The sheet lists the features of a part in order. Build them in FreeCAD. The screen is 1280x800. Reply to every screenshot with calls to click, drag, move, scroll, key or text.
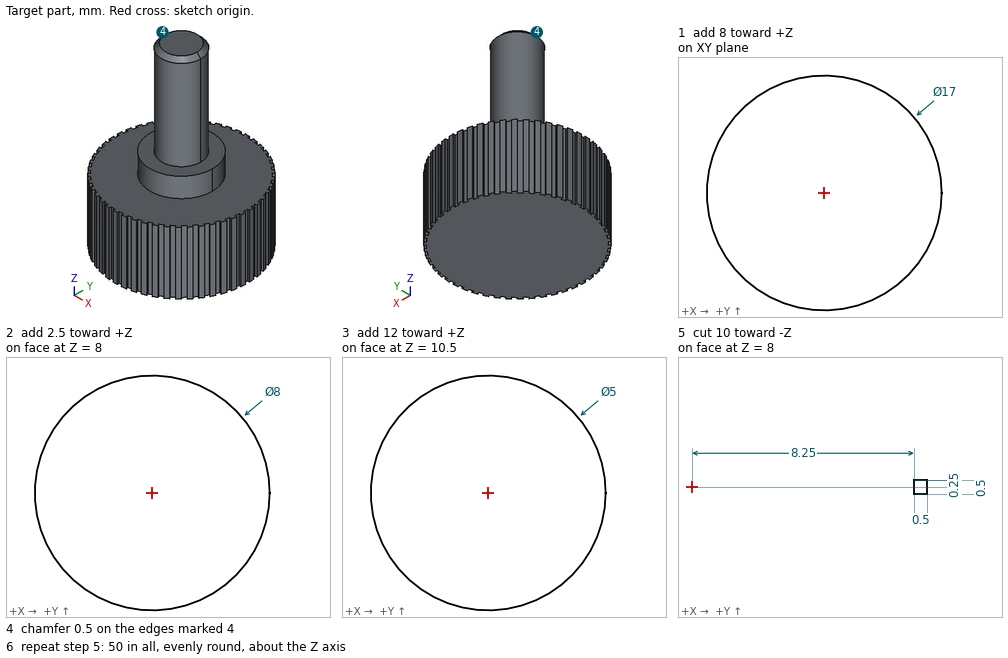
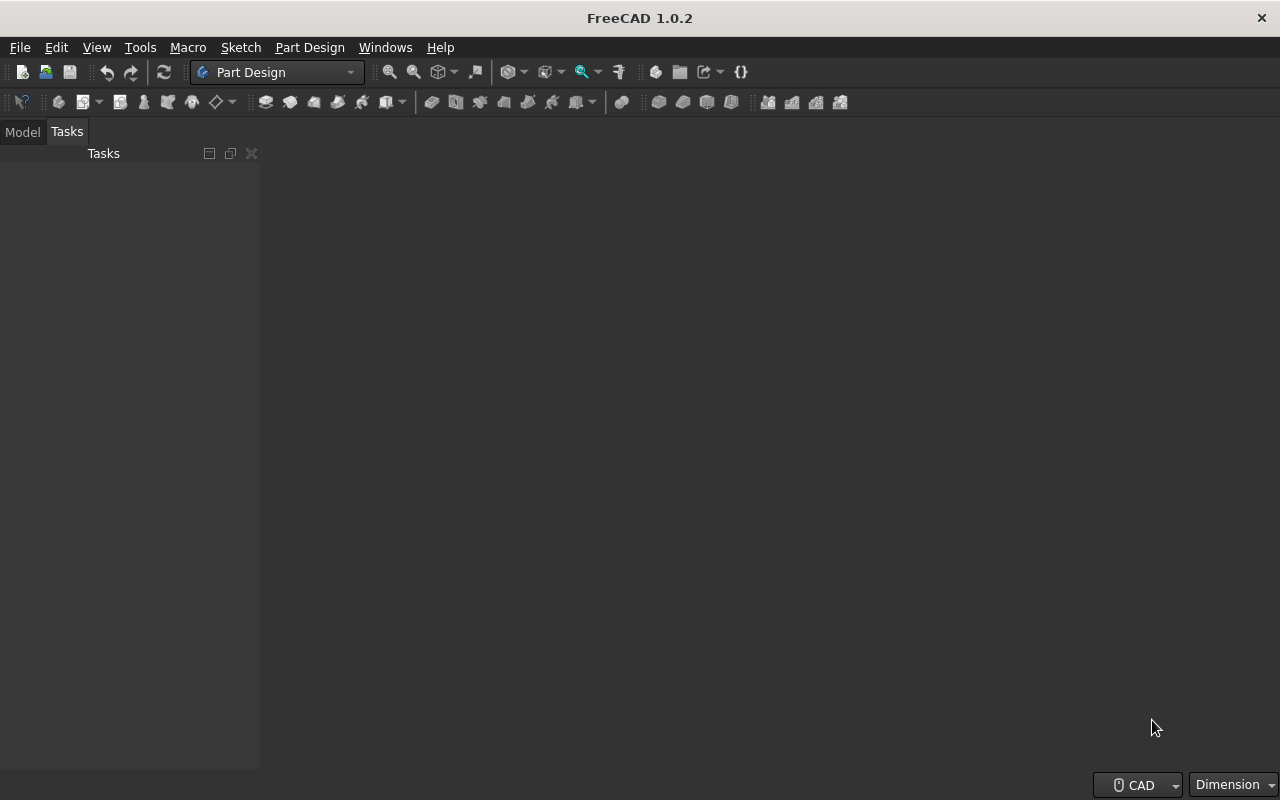
key(ctrl+n)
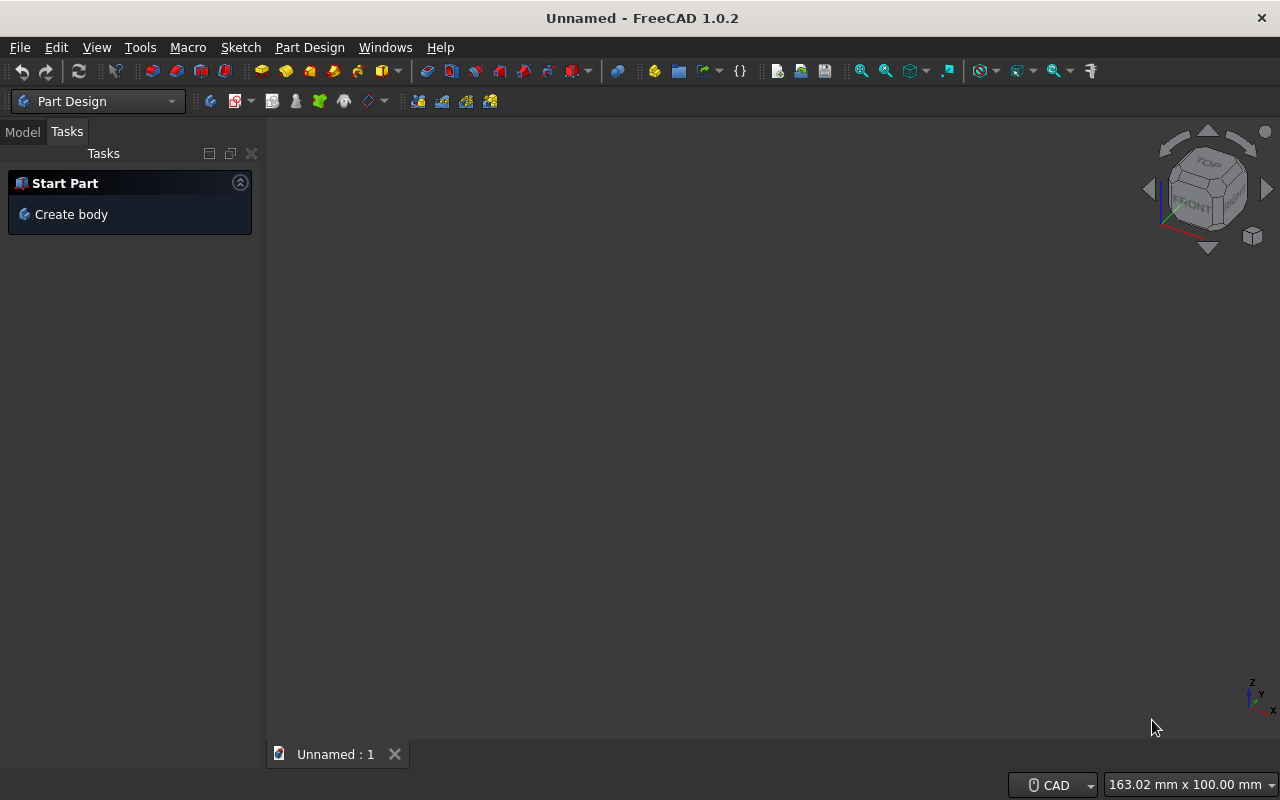
click(236, 102)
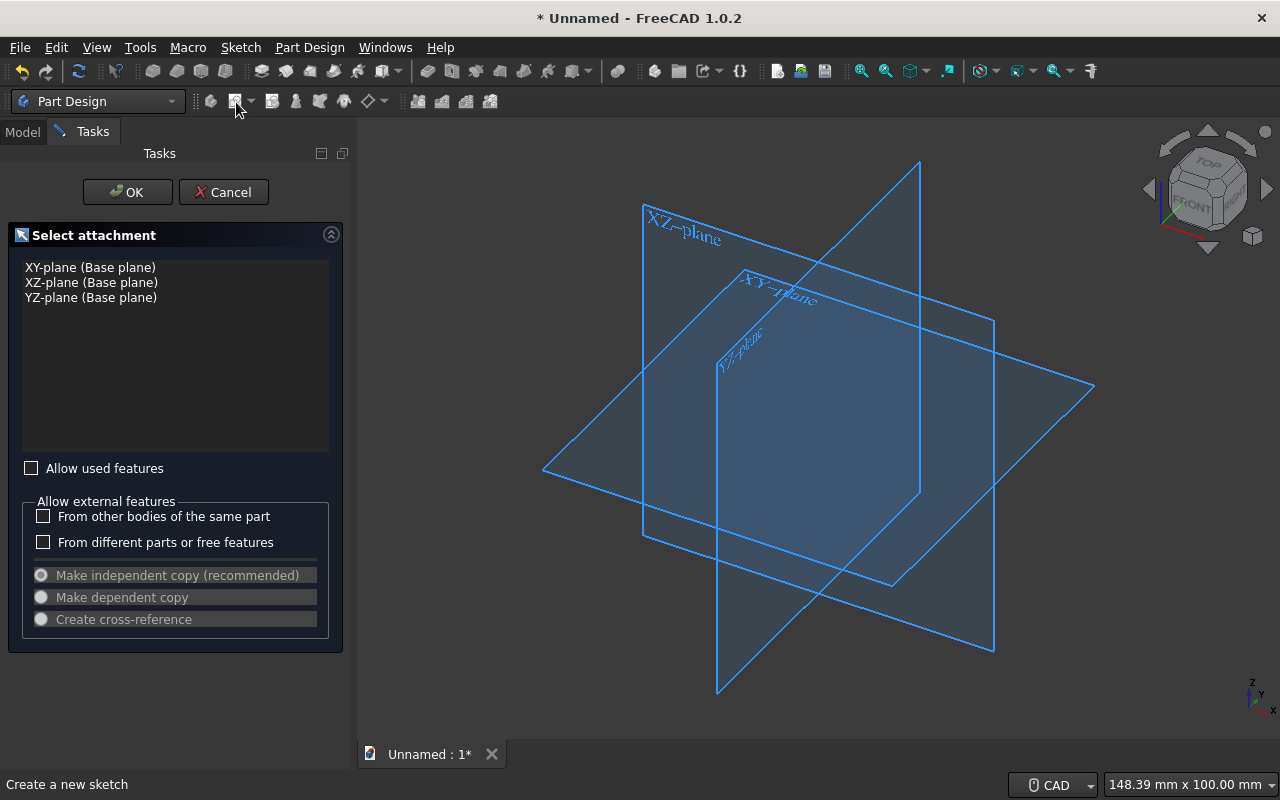
click(82, 268)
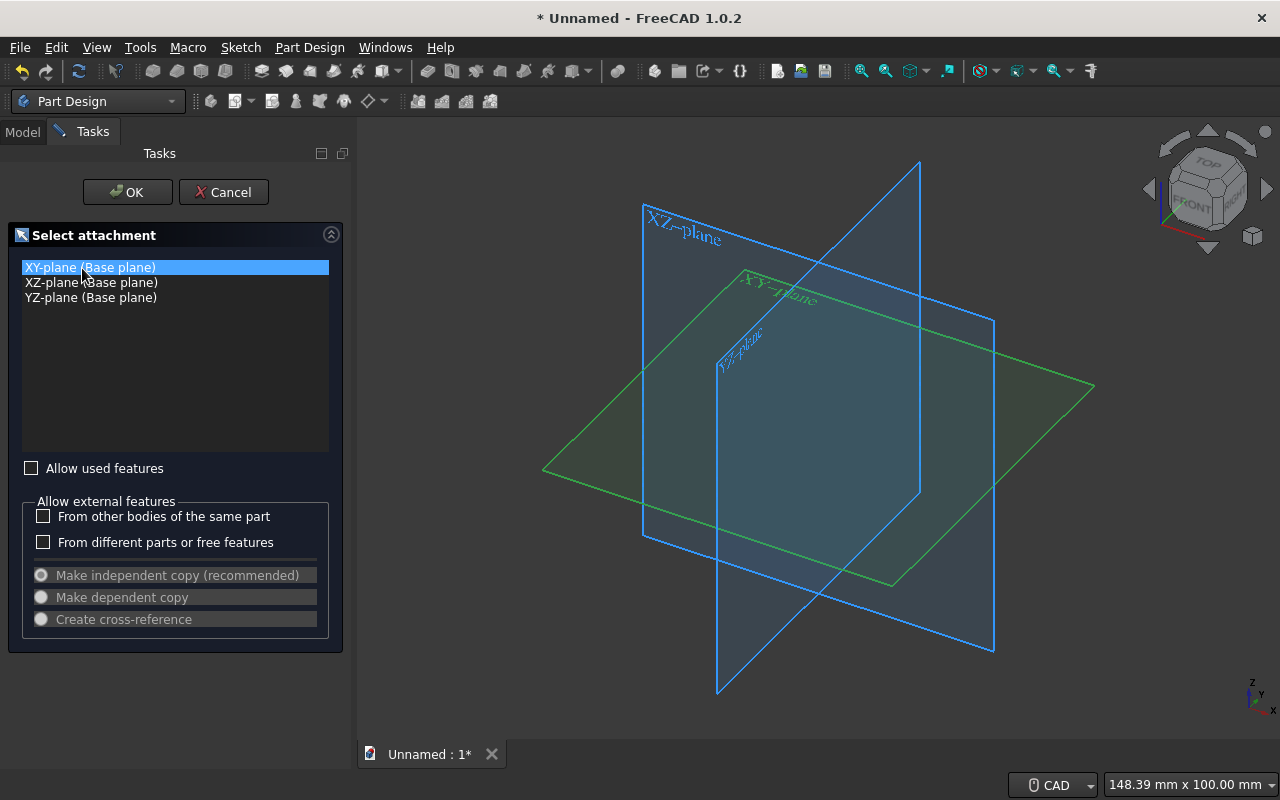
click(128, 192)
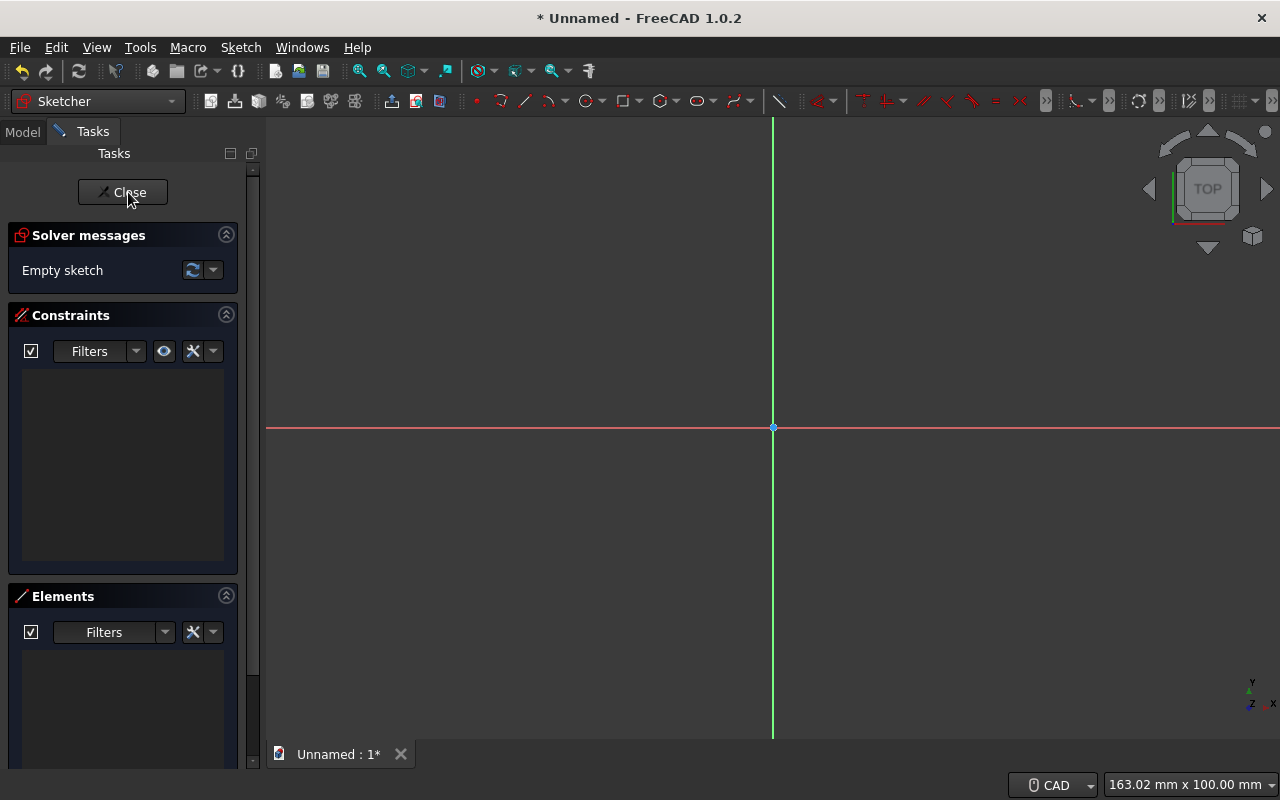
scroll(795, 428, up, 7)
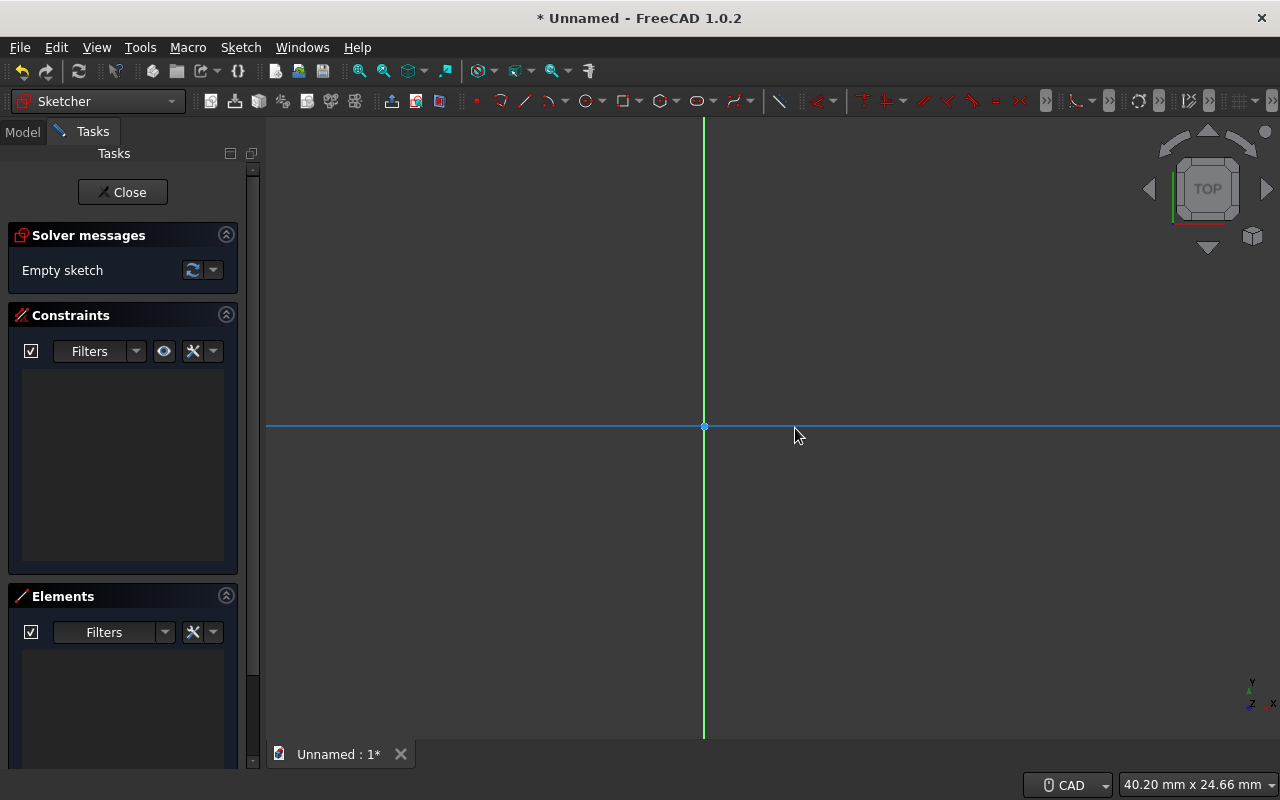
key(g)
key(c)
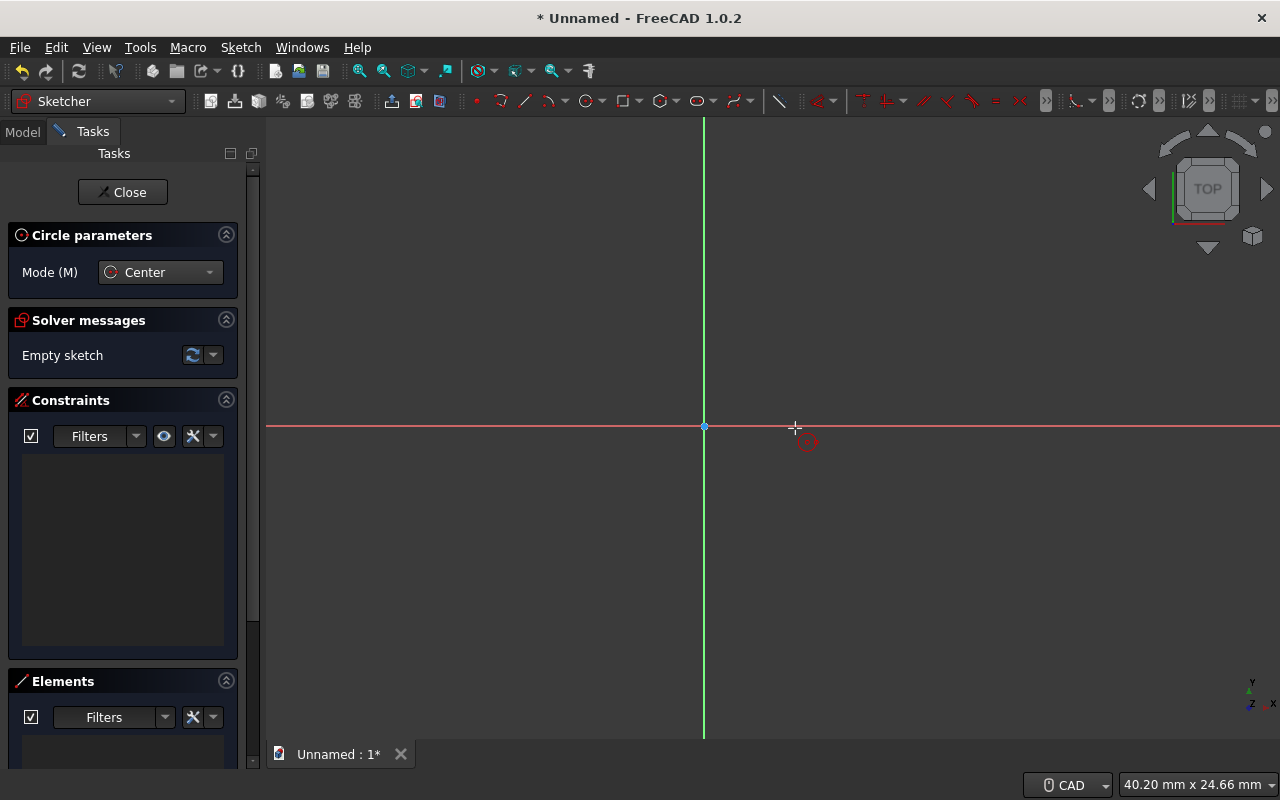
click(704, 426)
click(856, 275)
key(Escape)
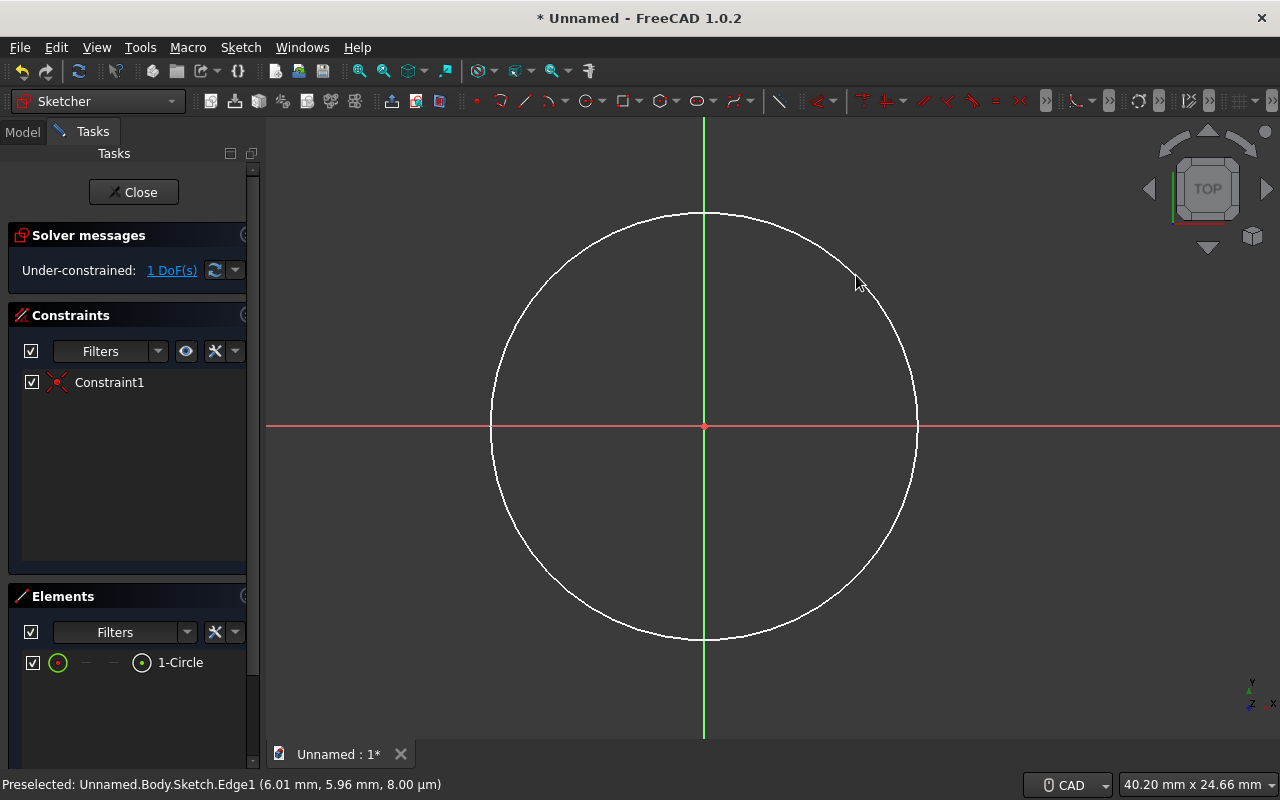
click(818, 102)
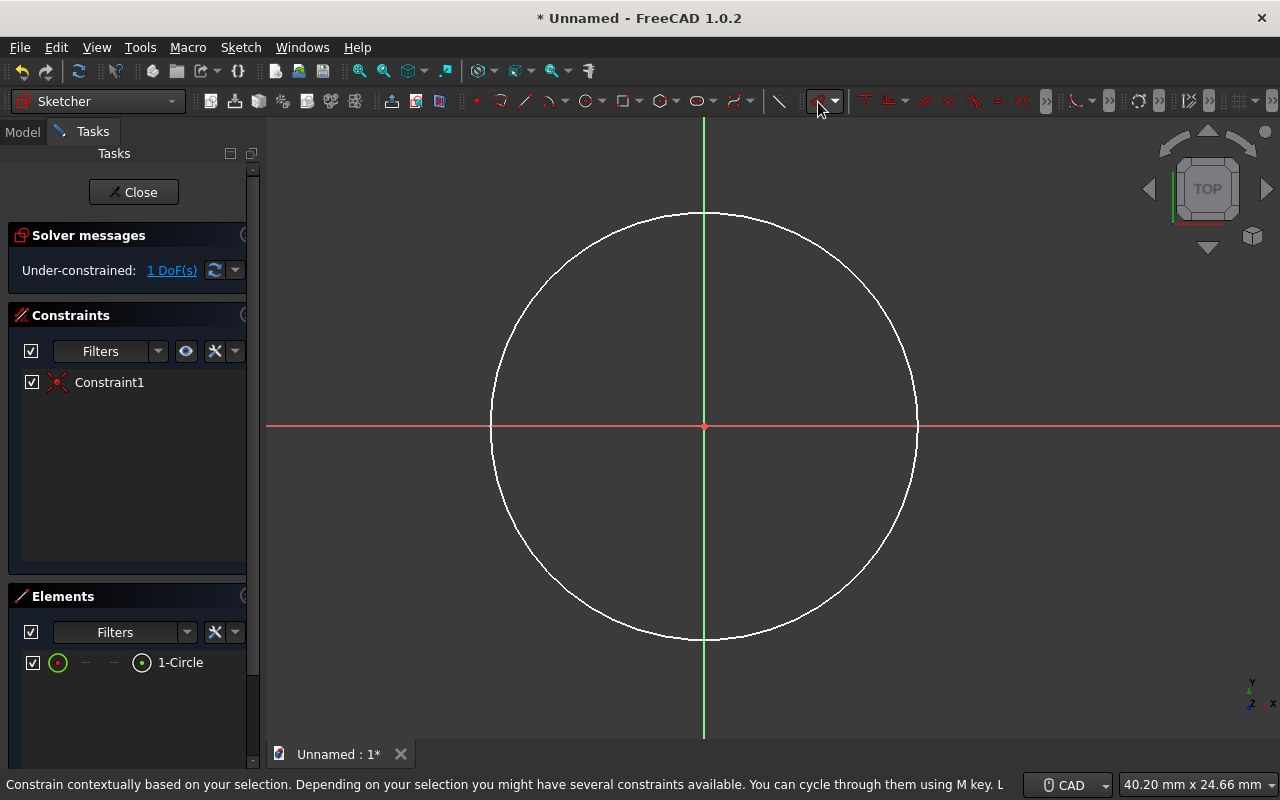
click(855, 275)
click(878, 252)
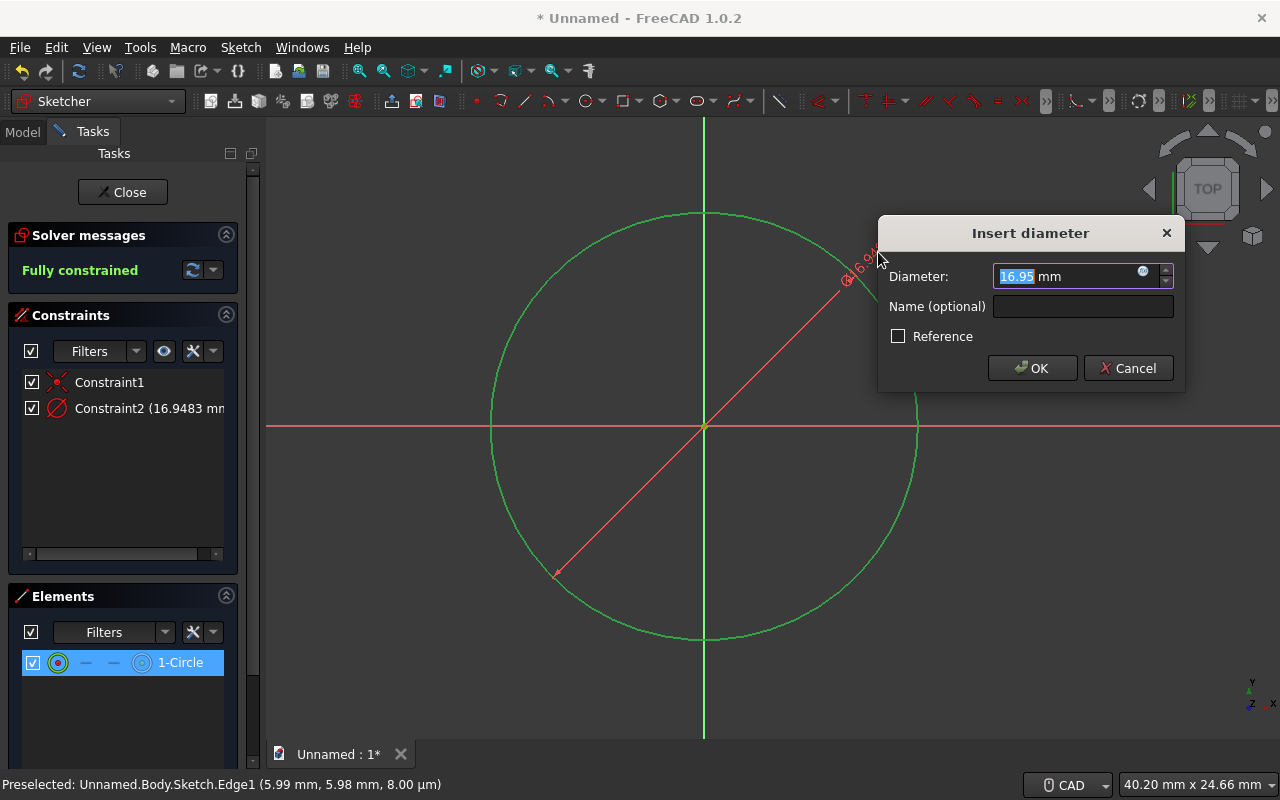
text(17)
key(Return)
key(Escape)